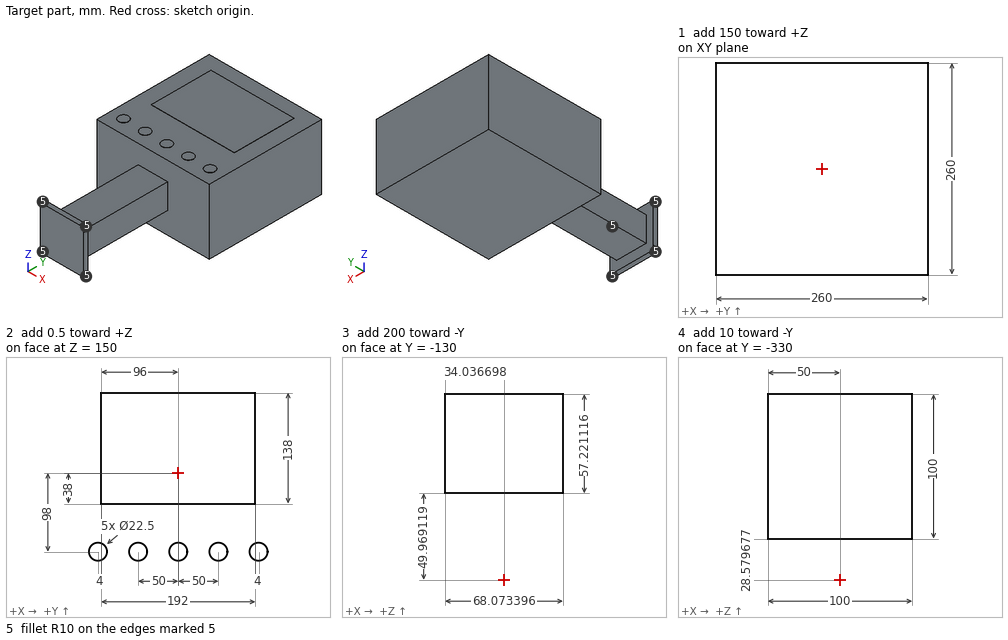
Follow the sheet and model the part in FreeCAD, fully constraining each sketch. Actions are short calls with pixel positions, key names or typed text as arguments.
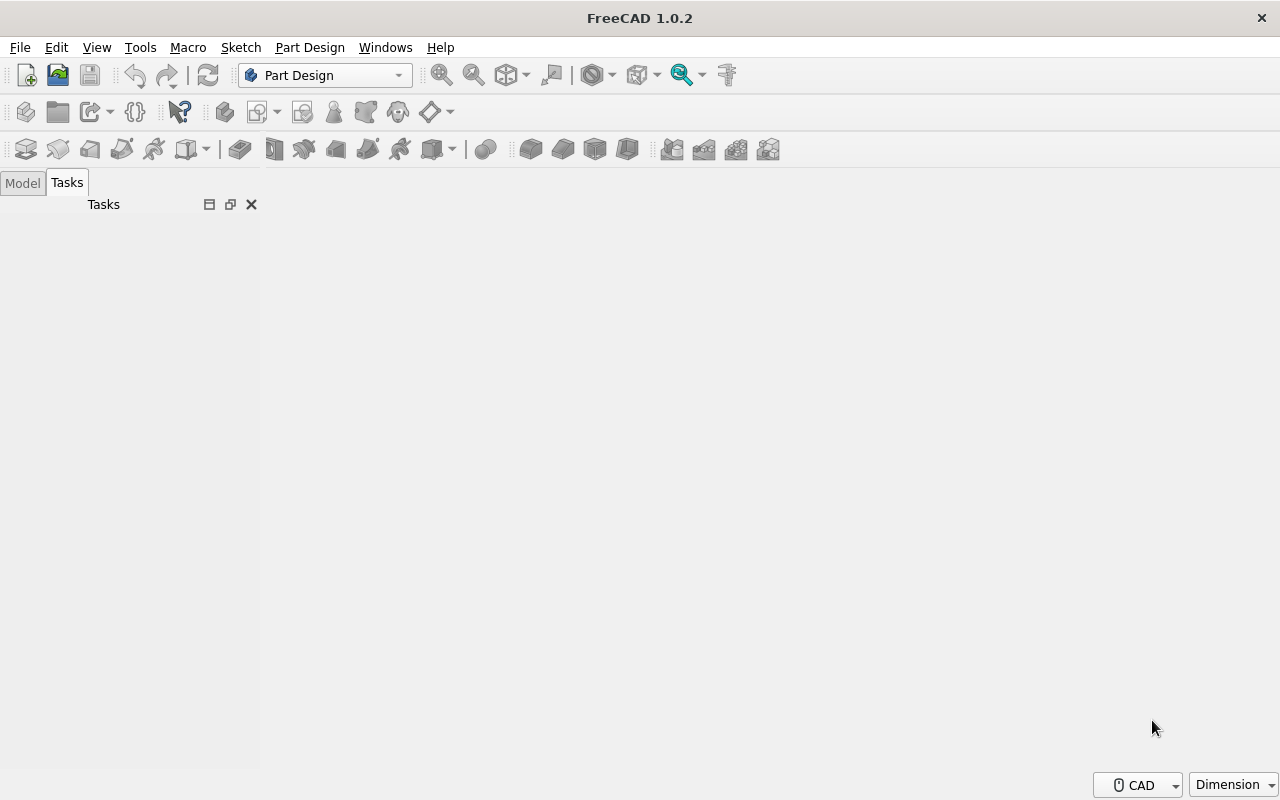
click(286, 76)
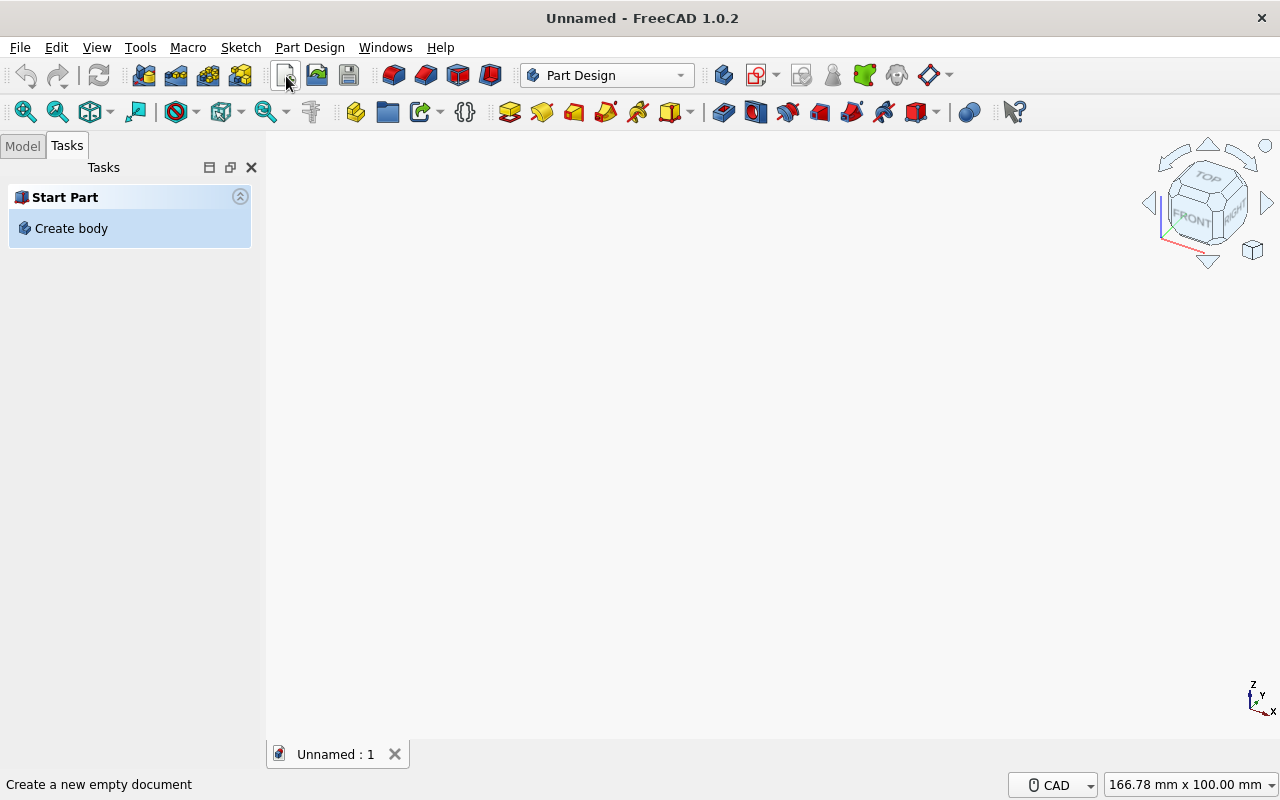
click(756, 76)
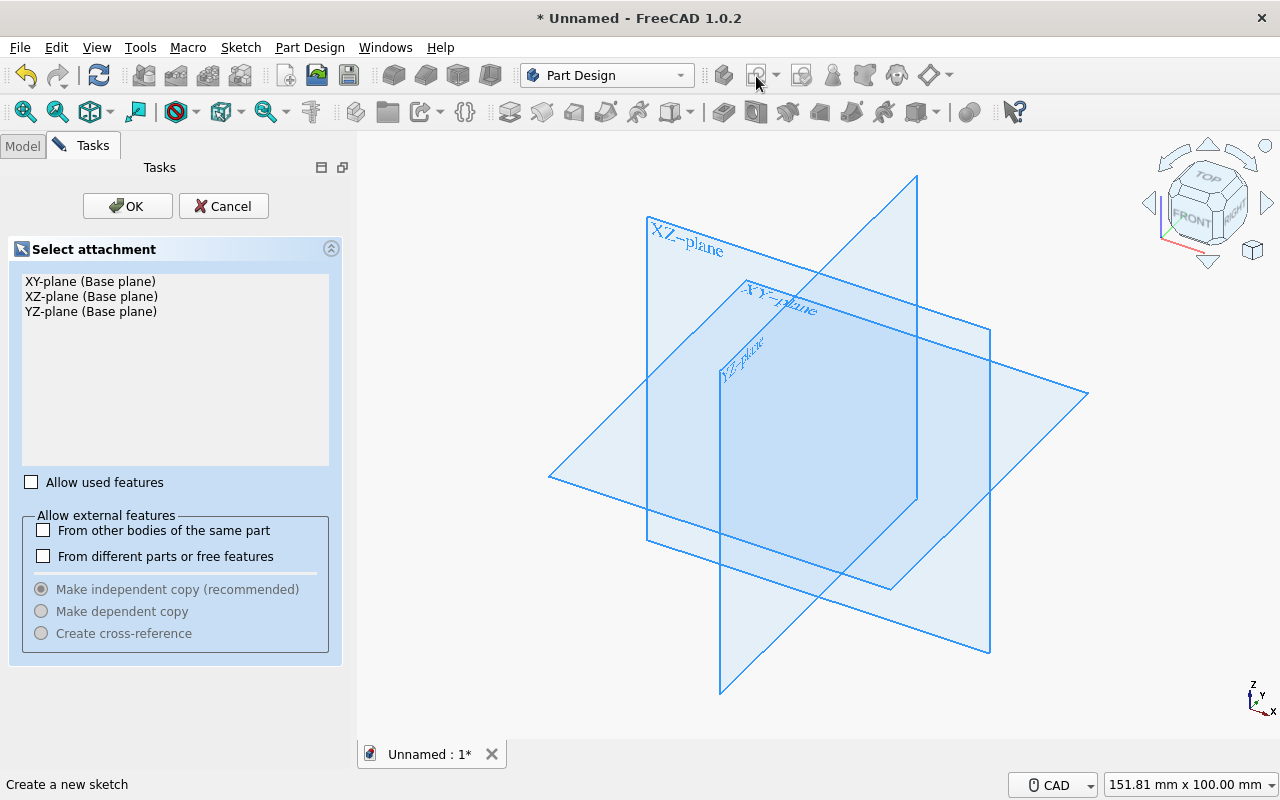
click(82, 282)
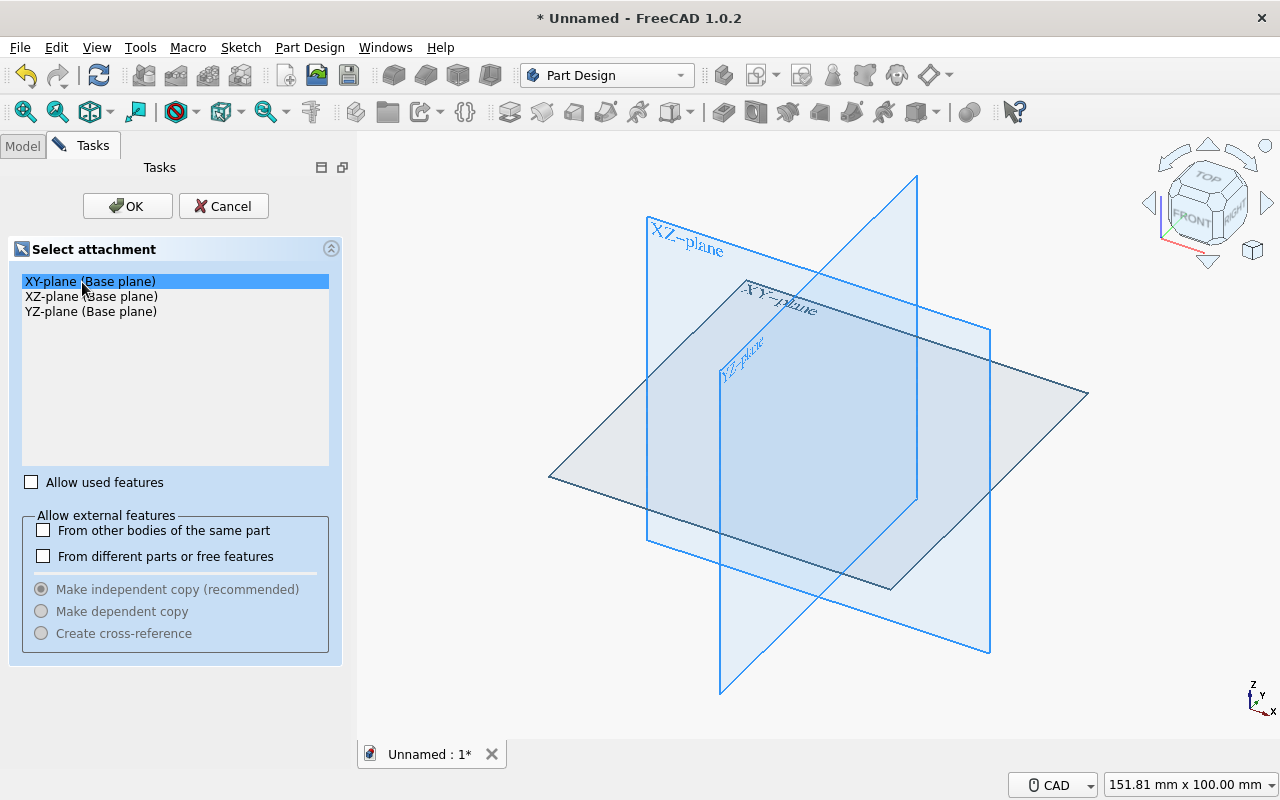
click(128, 206)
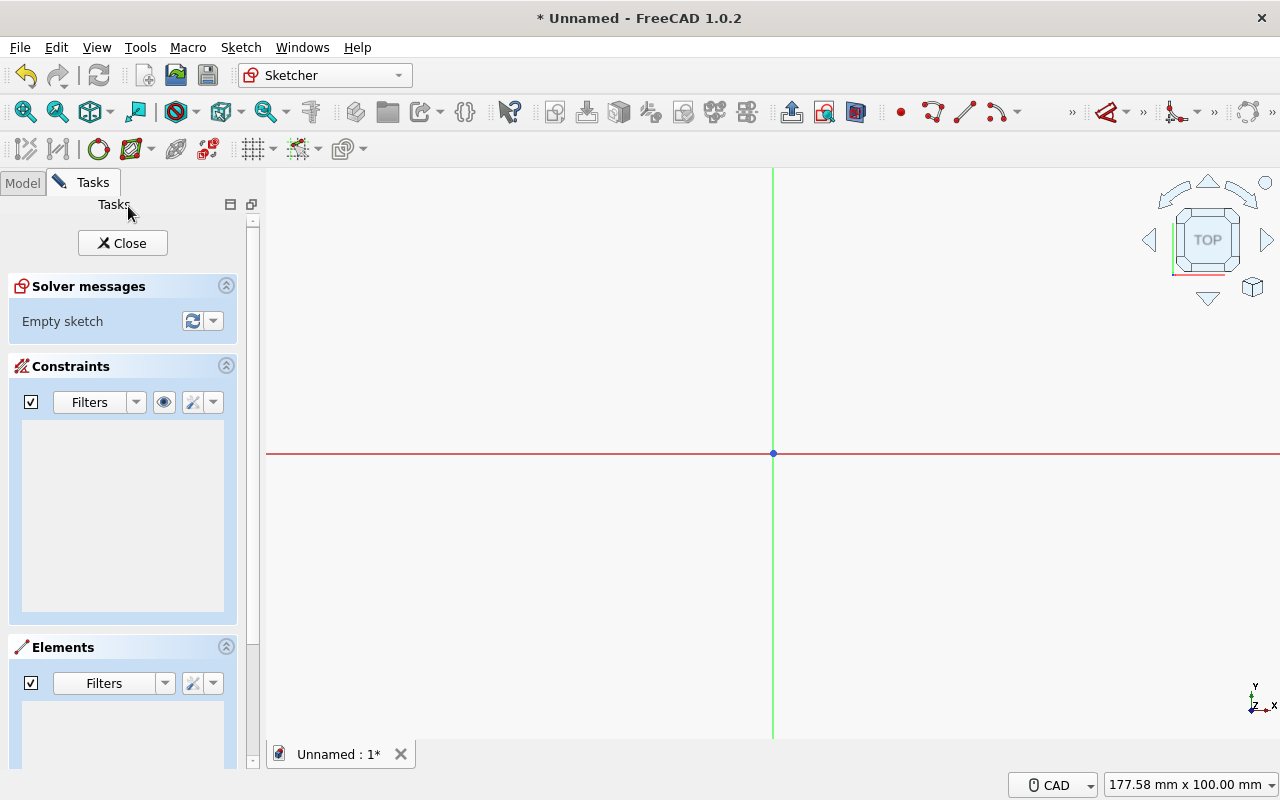
scroll(682, 454, down, 7)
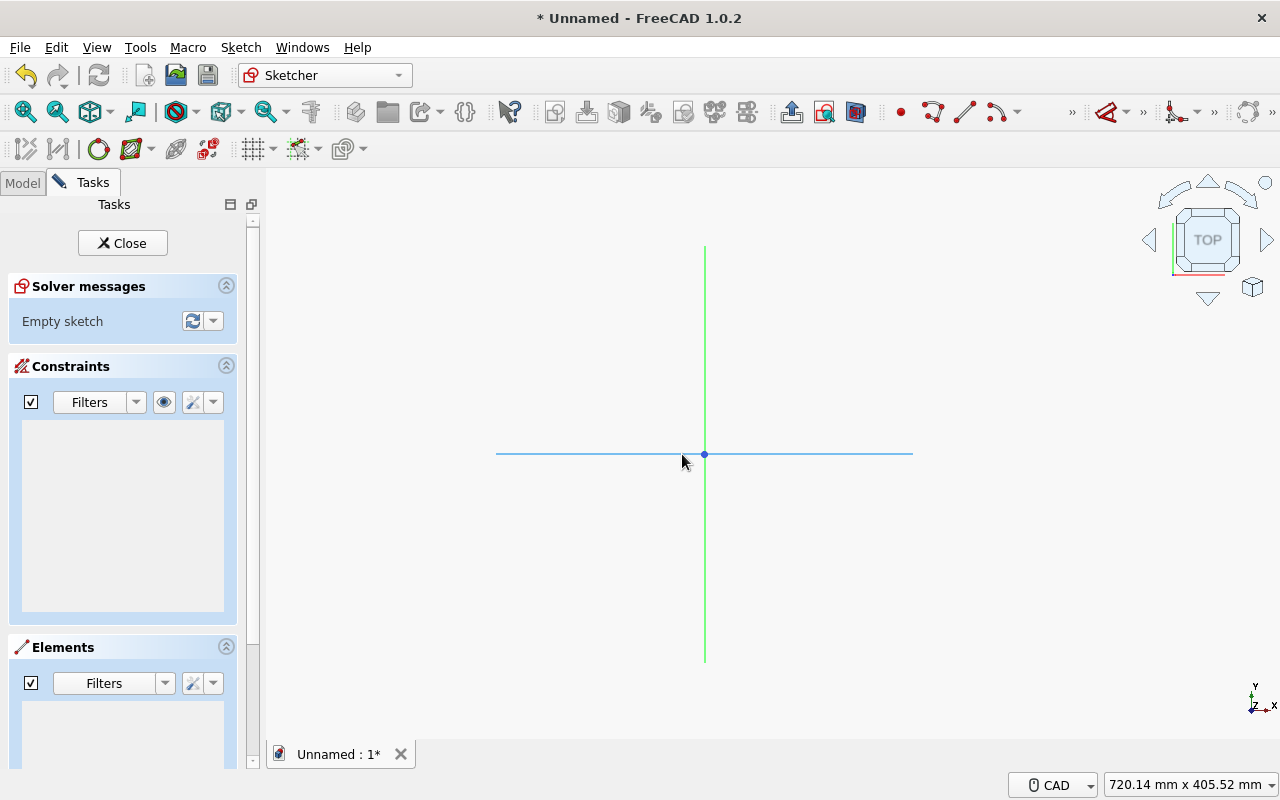
key(g)
key(v)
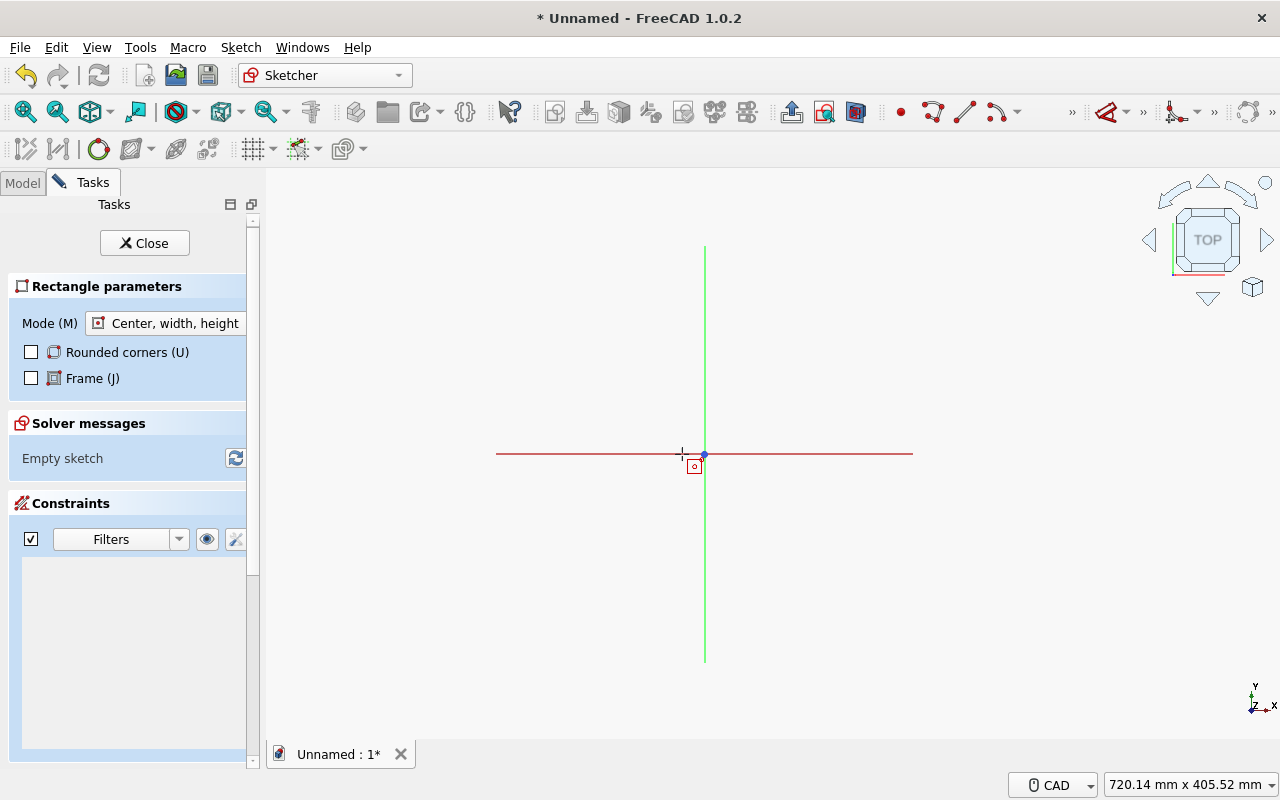
click(705, 454)
move(888, 271)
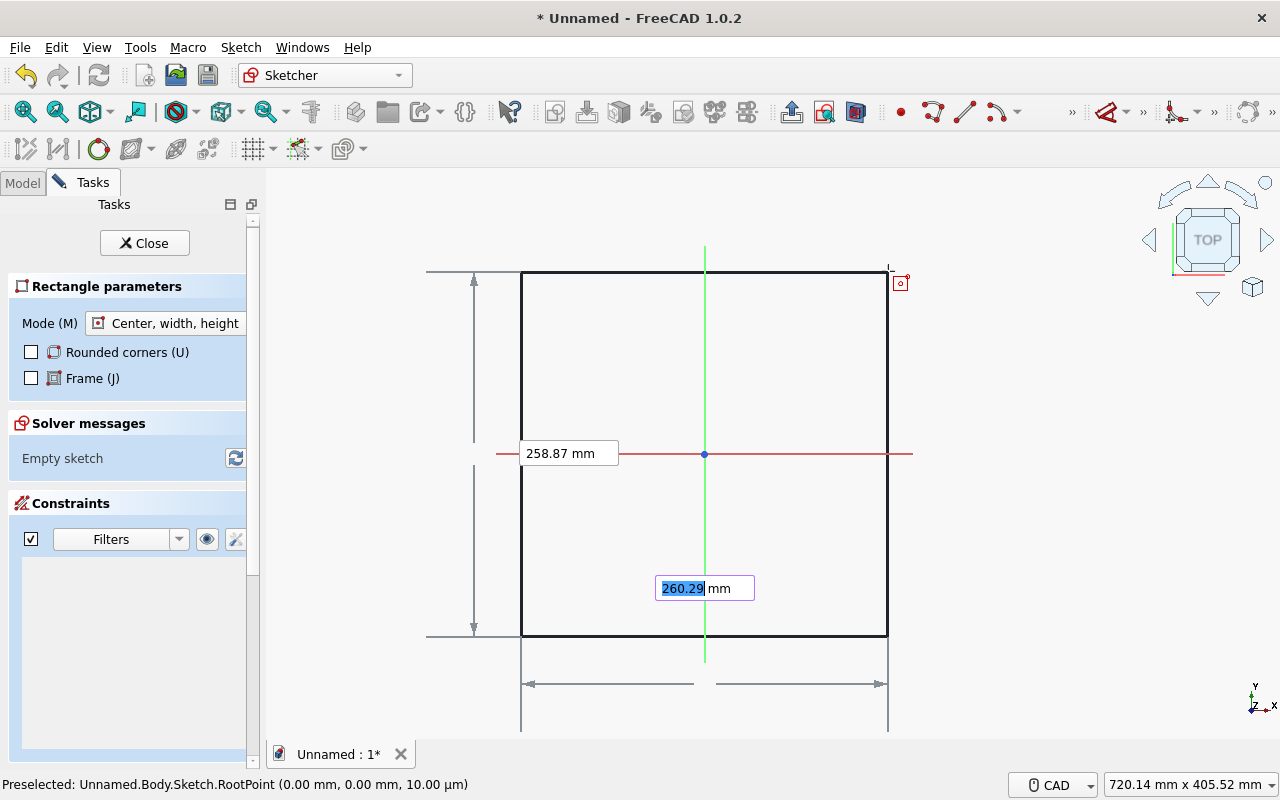
text(260)
key(Tab)
text(260)
key(Return)
key(Escape)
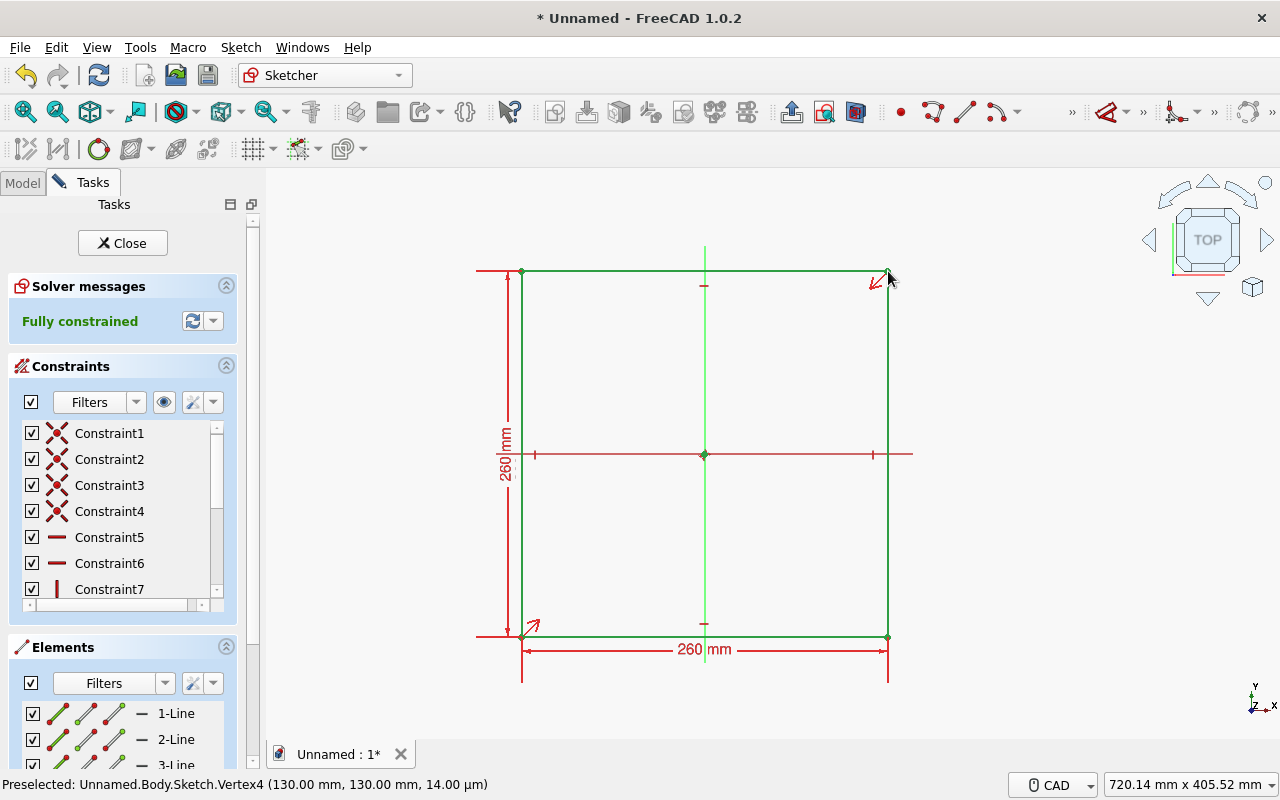
click(123, 243)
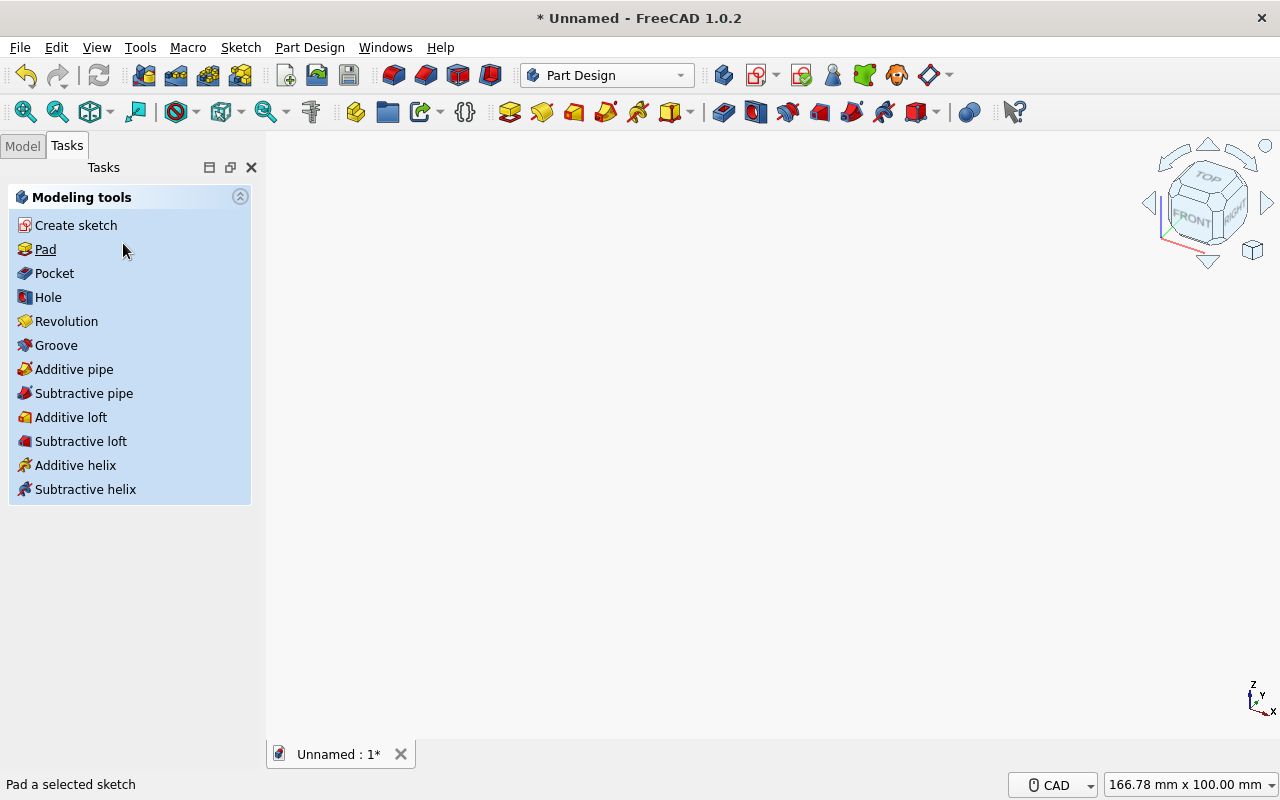
click(510, 112)